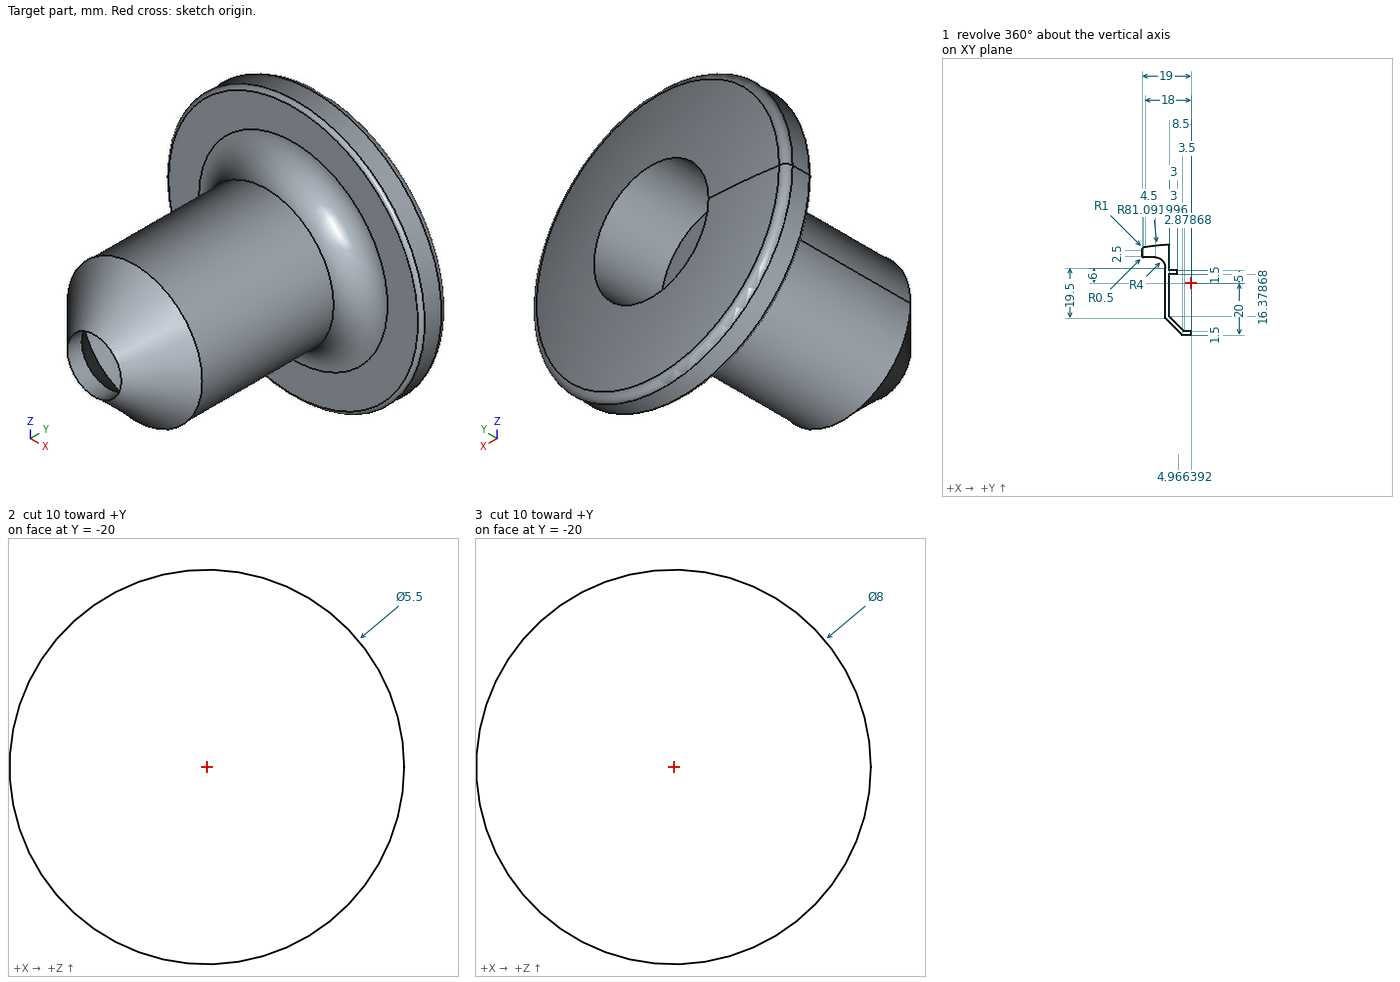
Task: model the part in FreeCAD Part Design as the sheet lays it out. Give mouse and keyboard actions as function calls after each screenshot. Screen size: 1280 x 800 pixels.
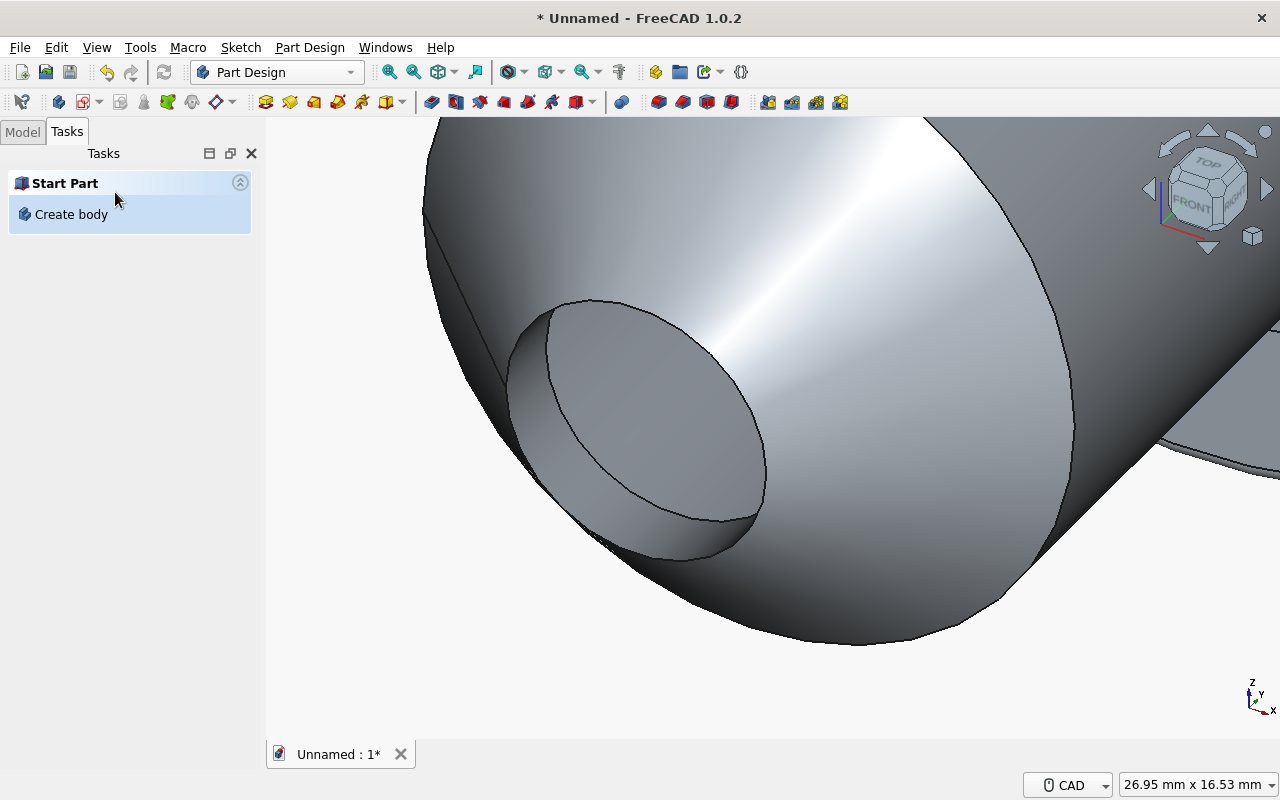
key(0)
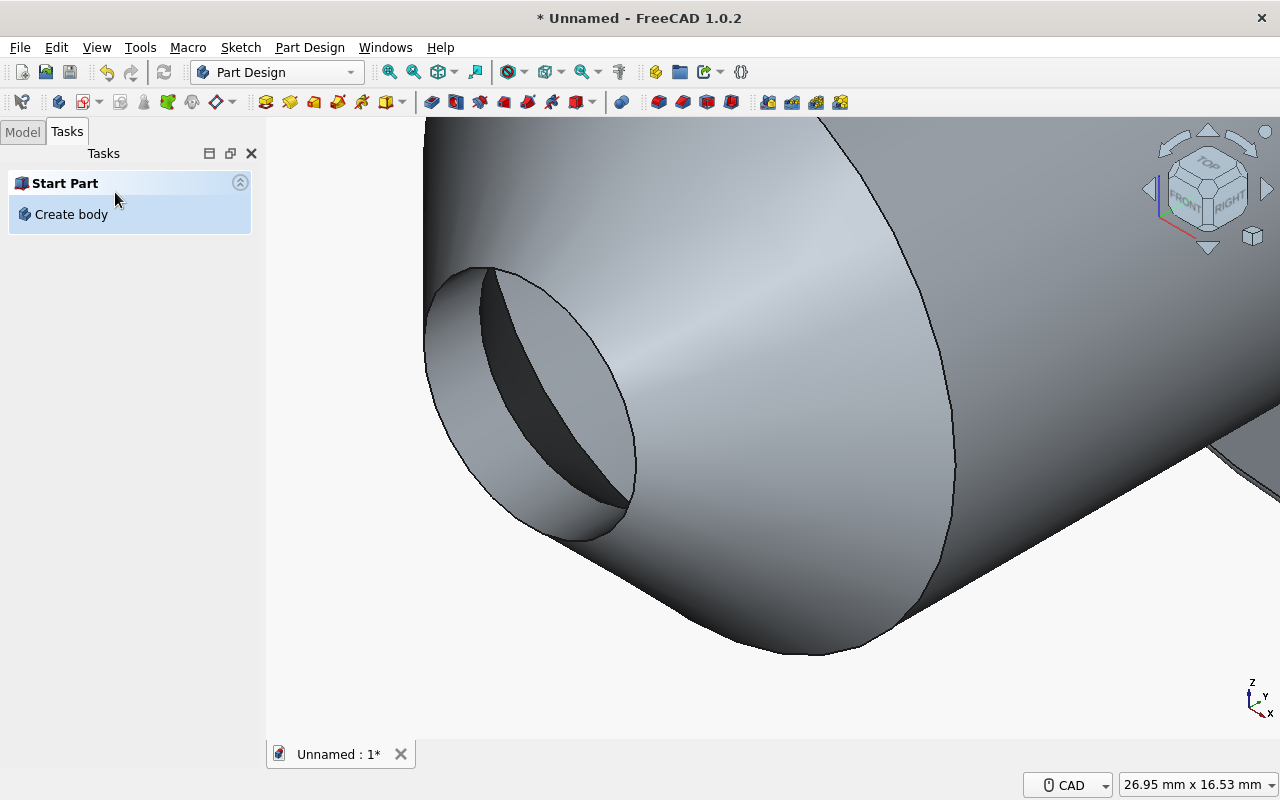
click(390, 72)